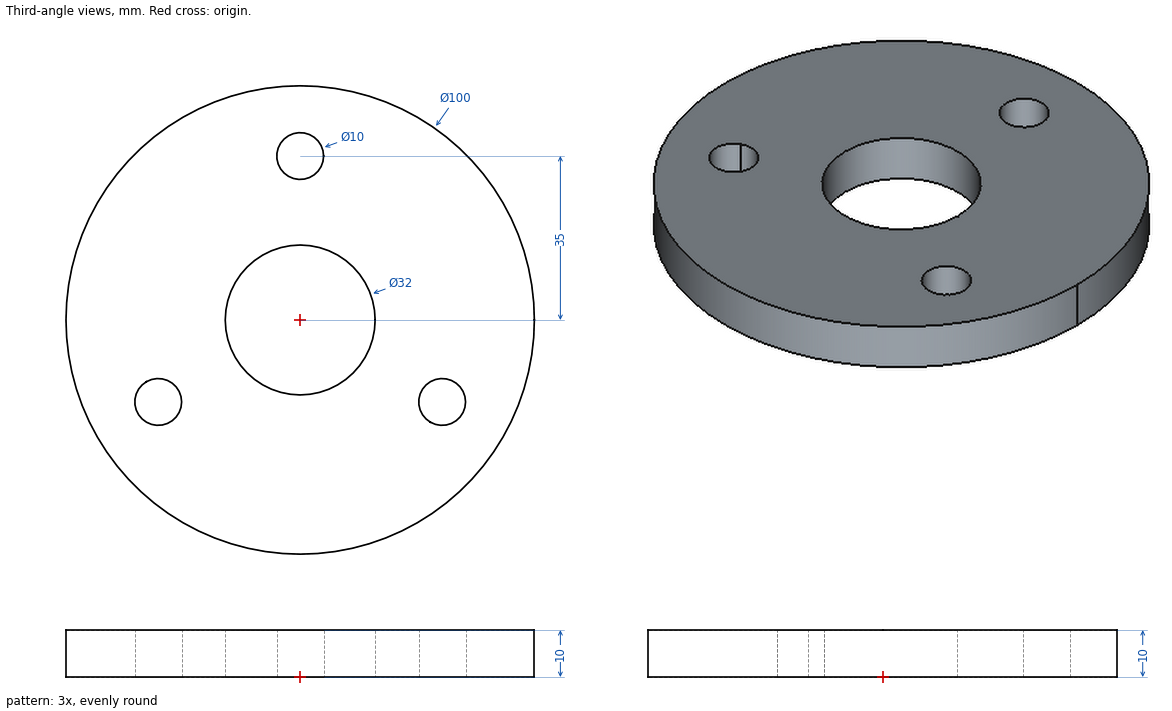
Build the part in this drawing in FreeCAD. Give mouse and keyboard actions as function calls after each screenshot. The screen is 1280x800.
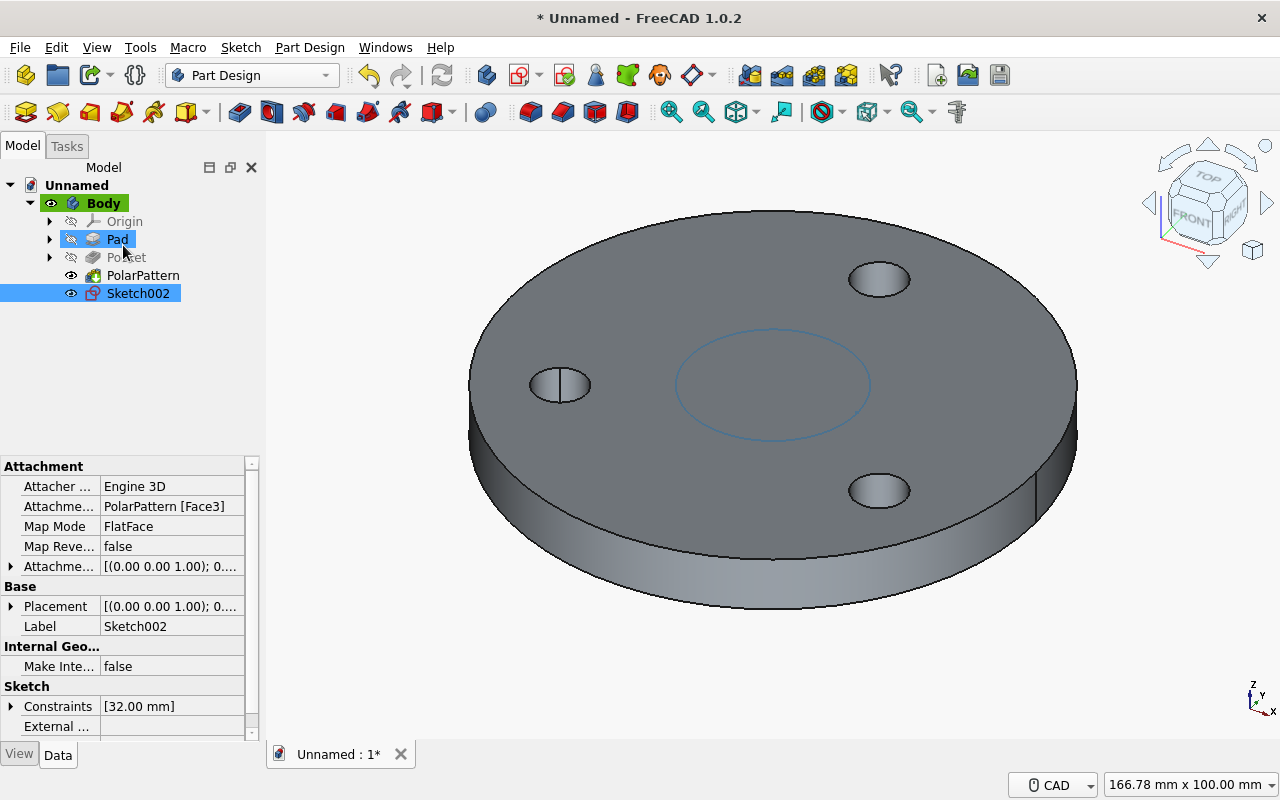
click(240, 112)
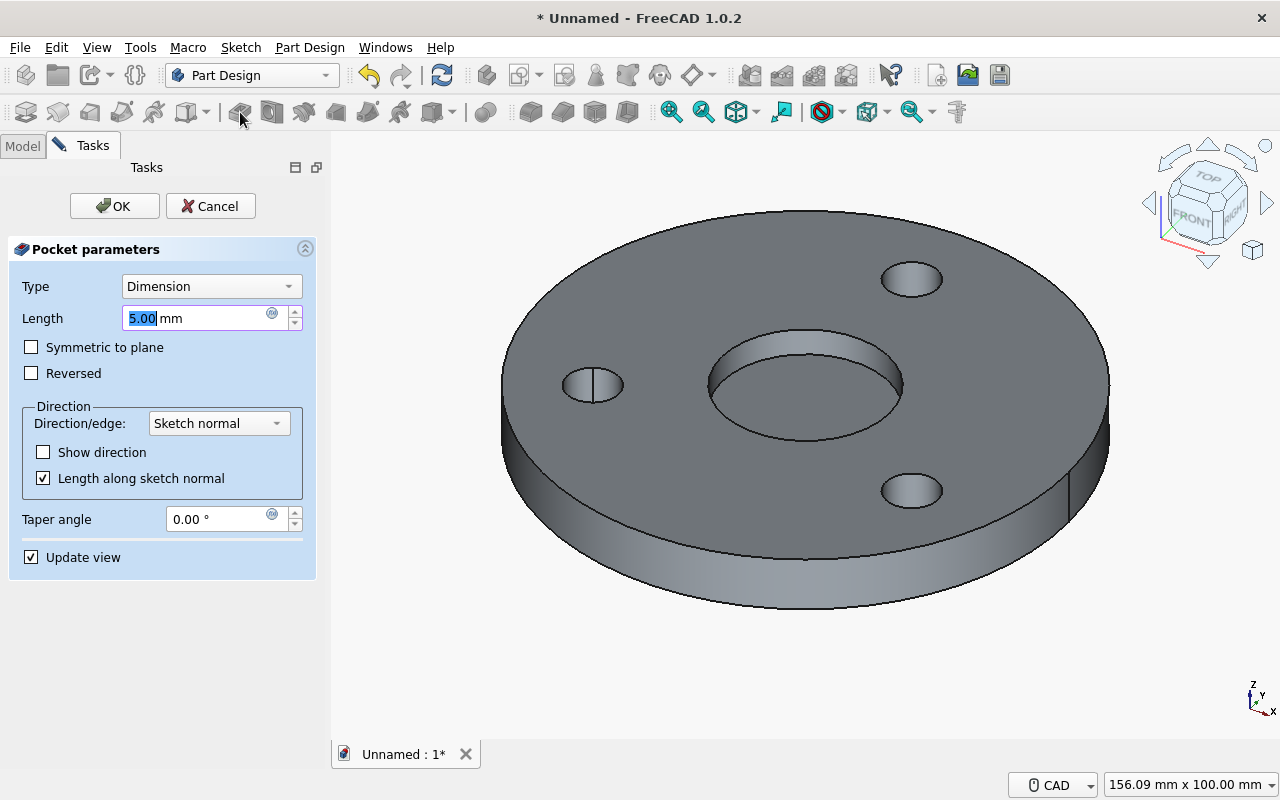
text(10)
key(Tab)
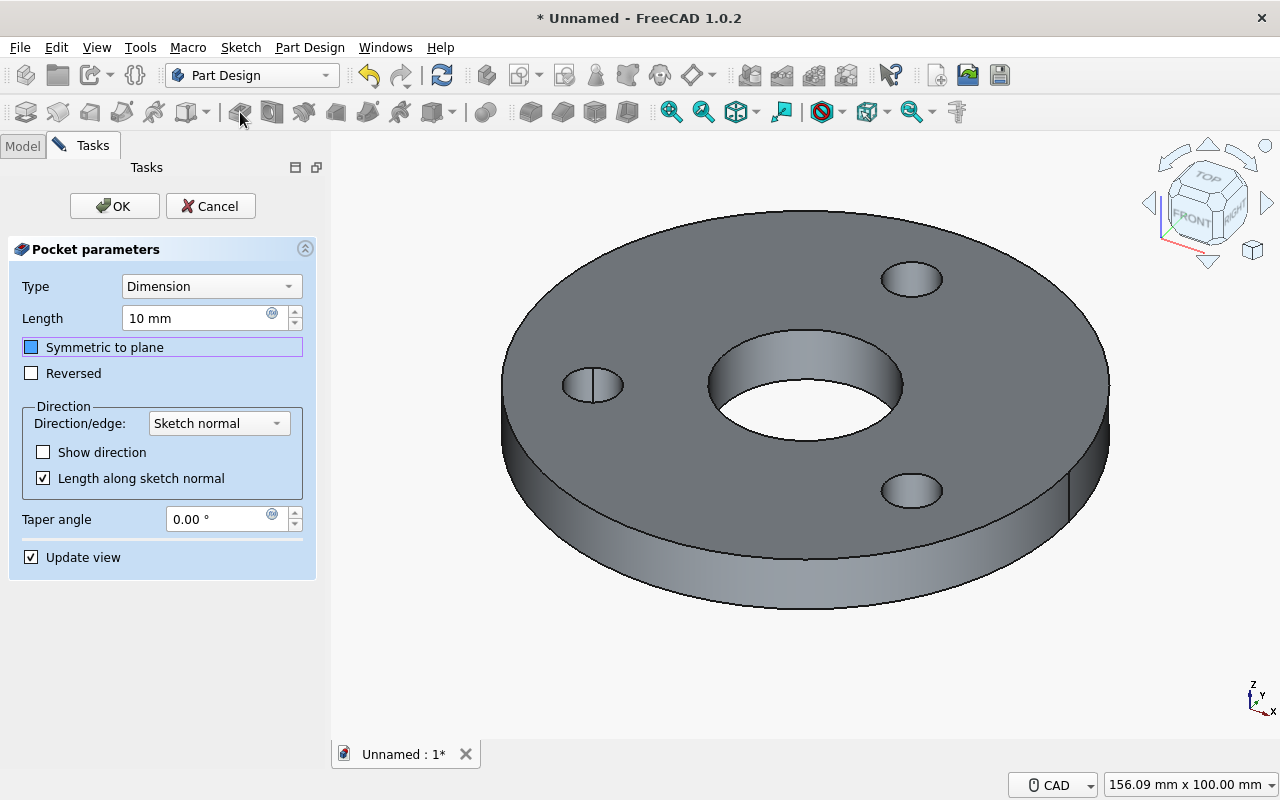
click(115, 206)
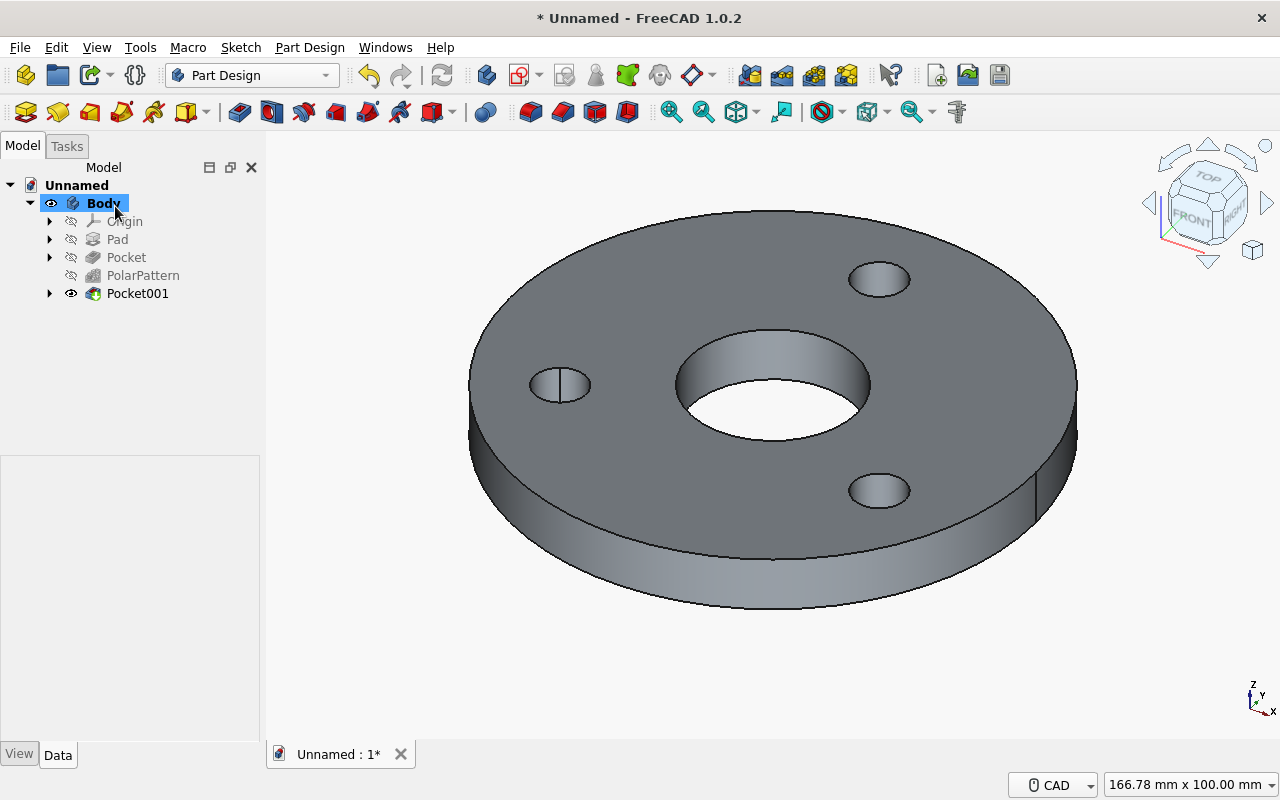
key(0)